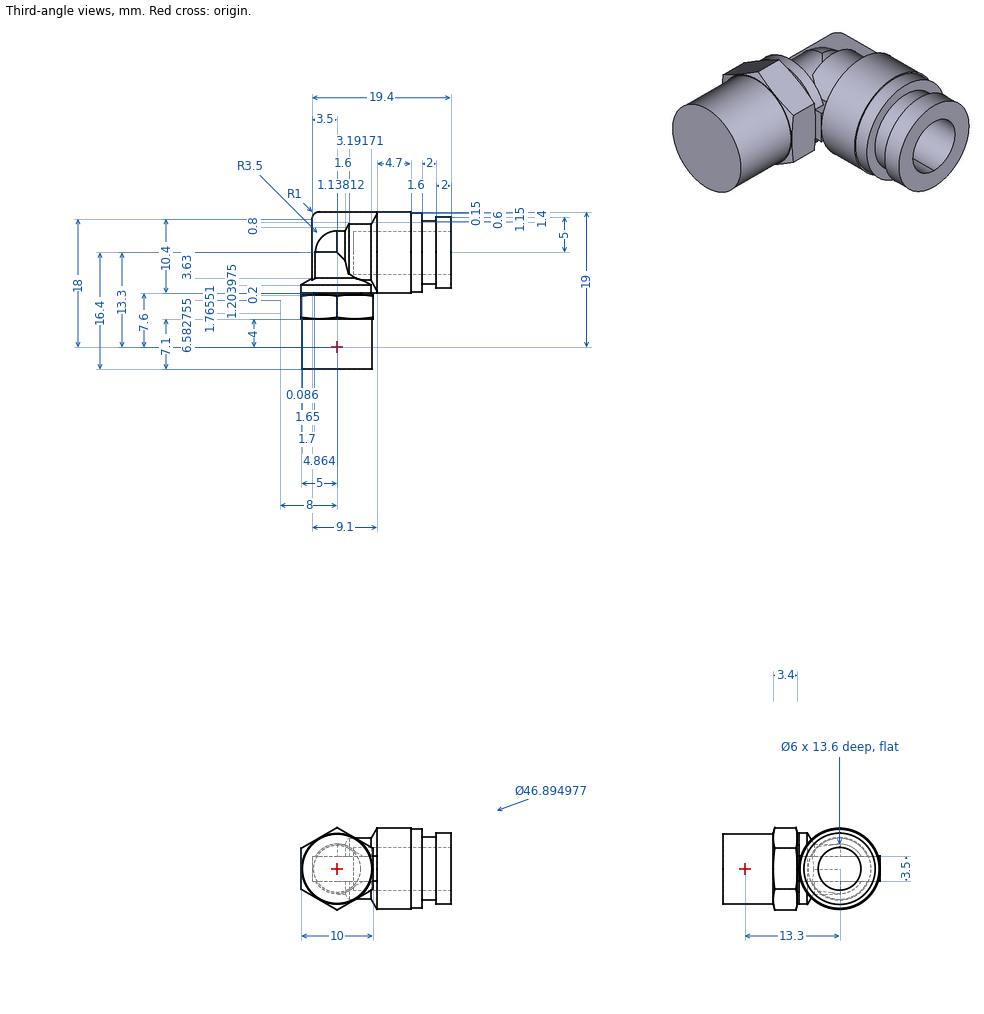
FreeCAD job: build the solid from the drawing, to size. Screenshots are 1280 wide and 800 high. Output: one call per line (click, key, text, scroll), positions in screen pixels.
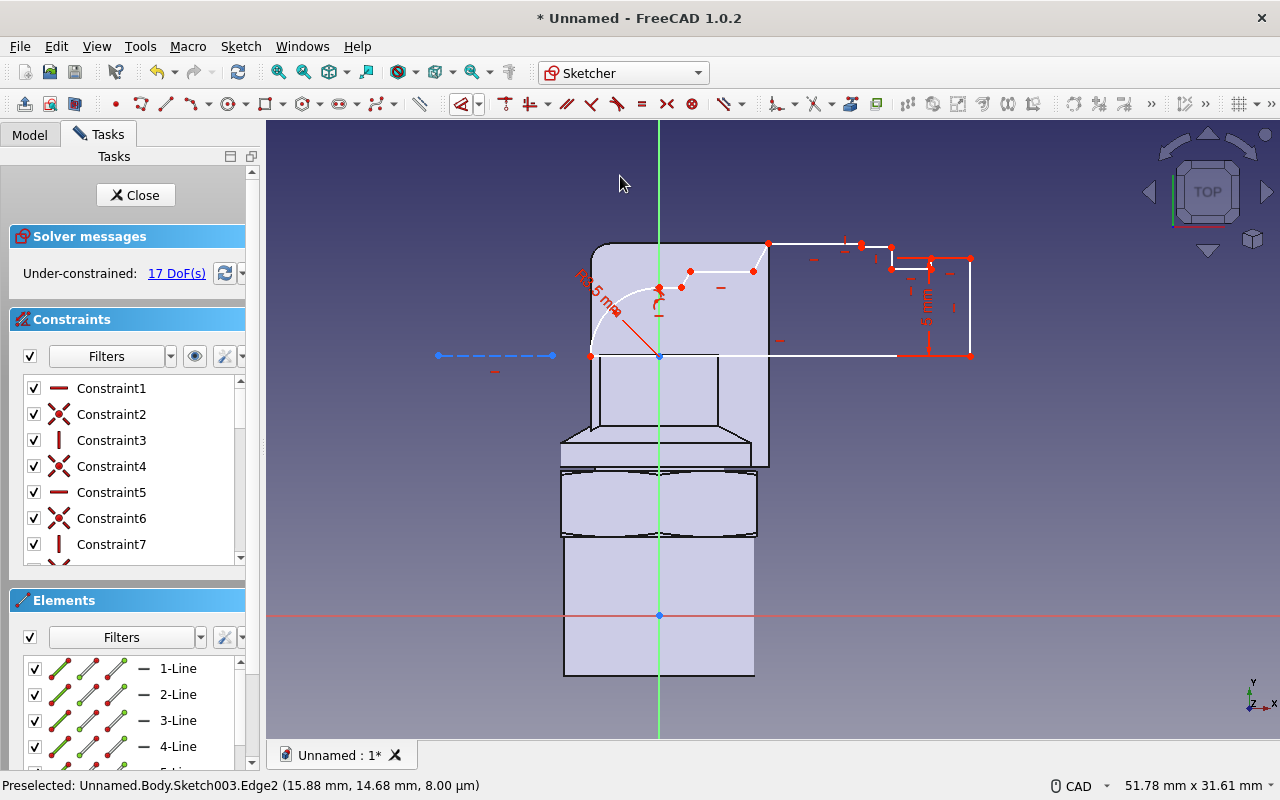
click(958, 258)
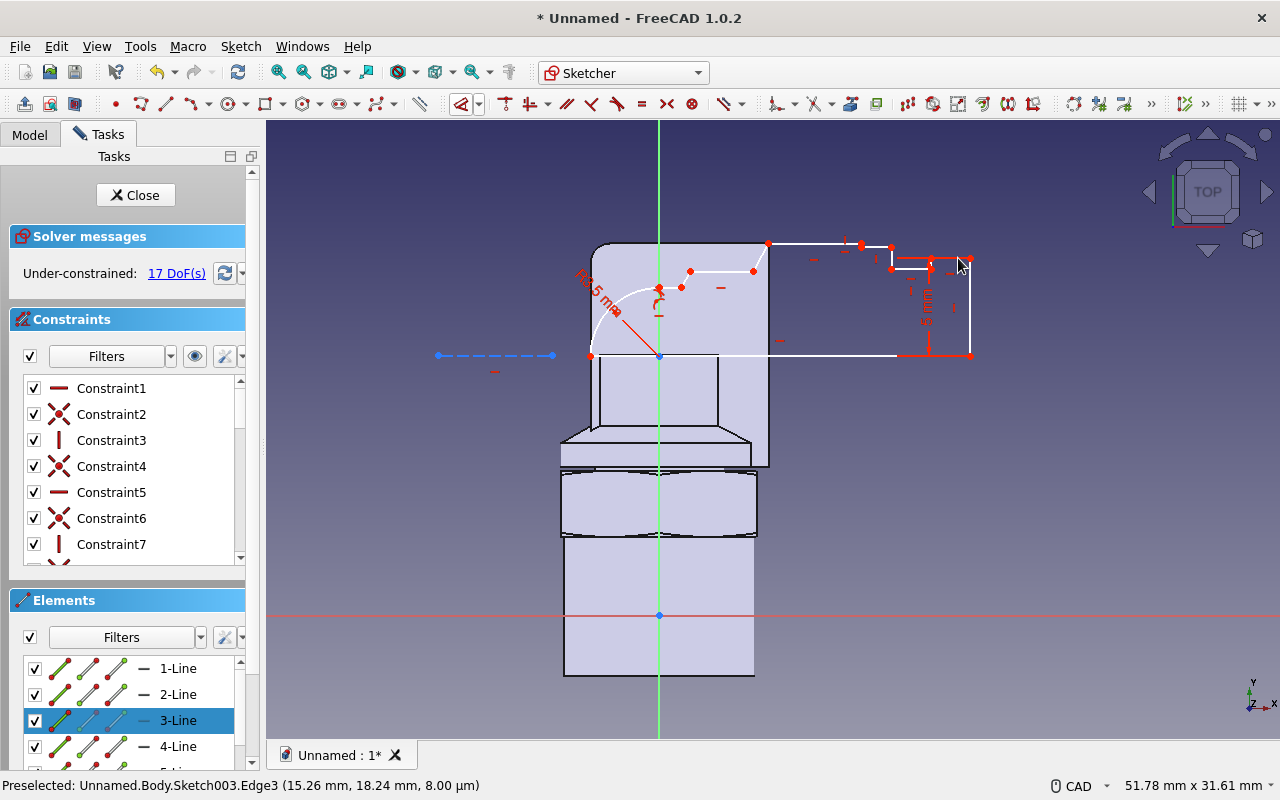
key(l)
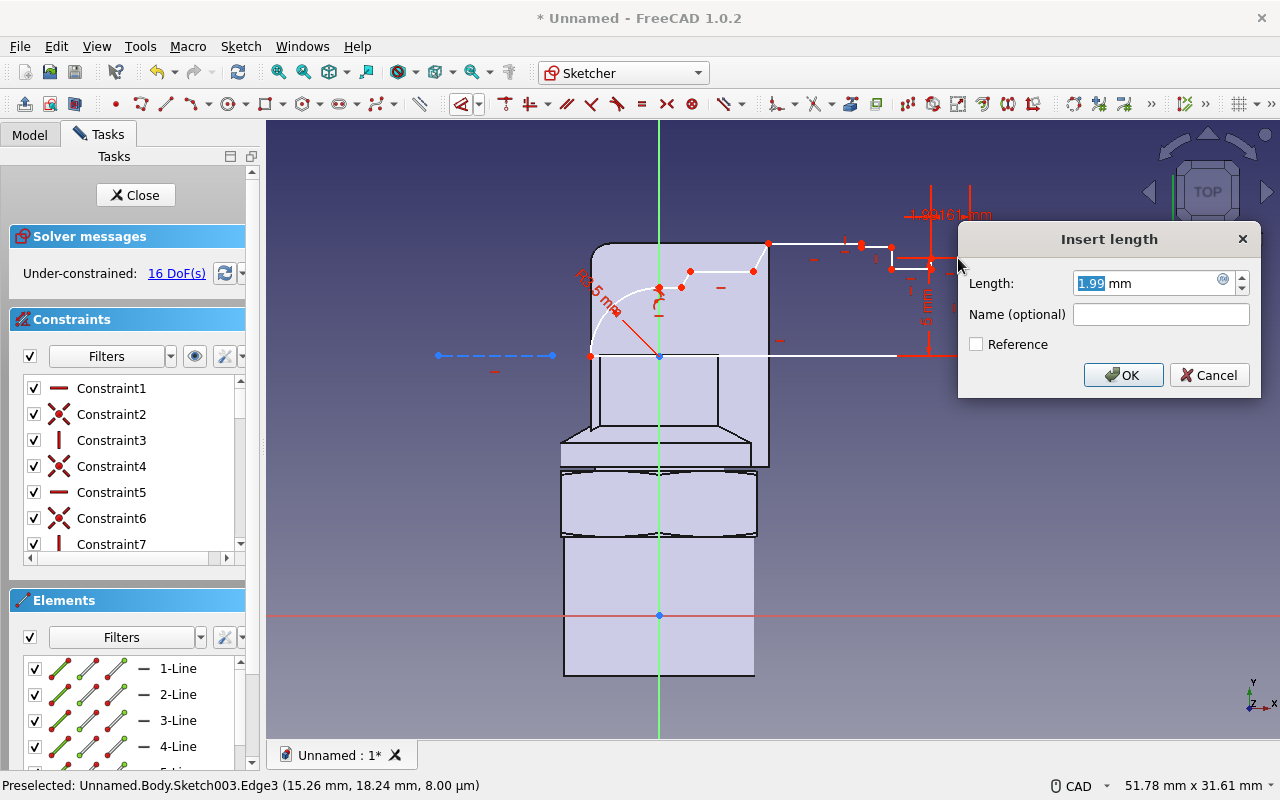
text(2)
key(Return)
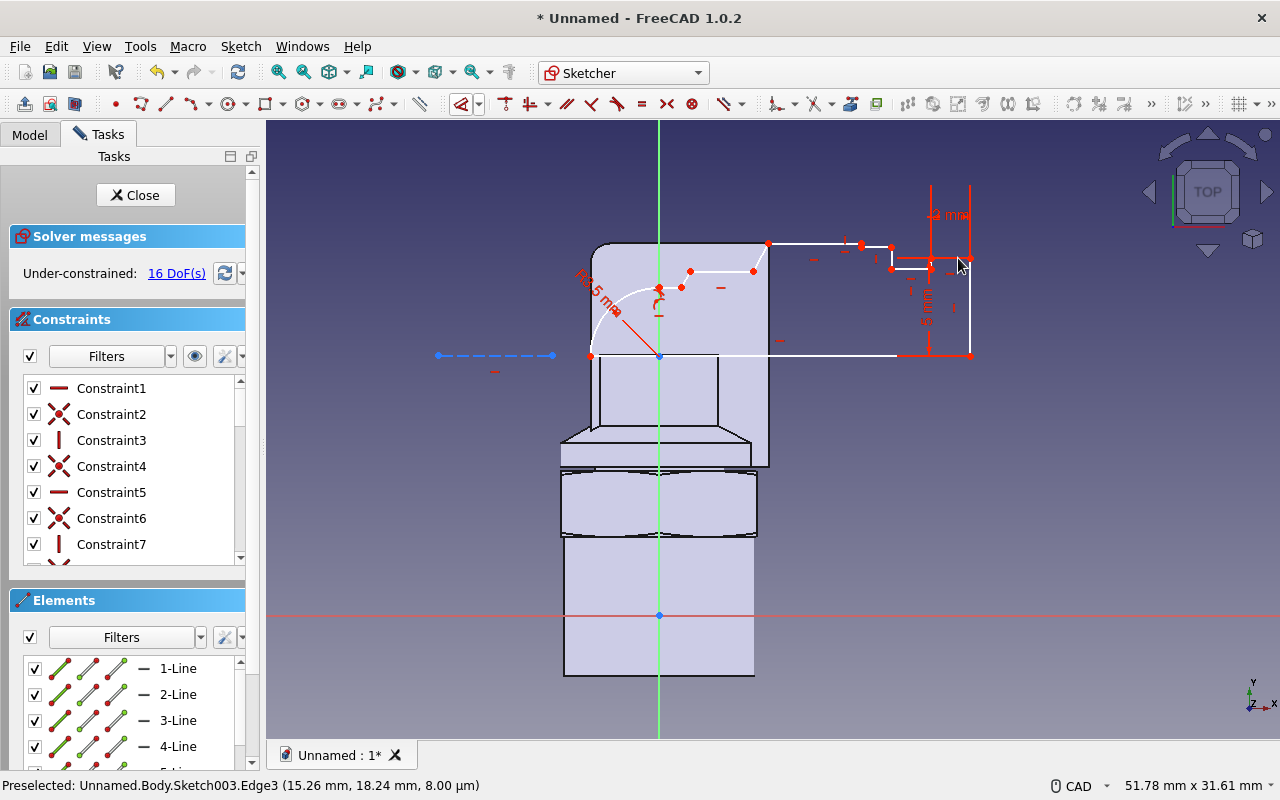
click(919, 269)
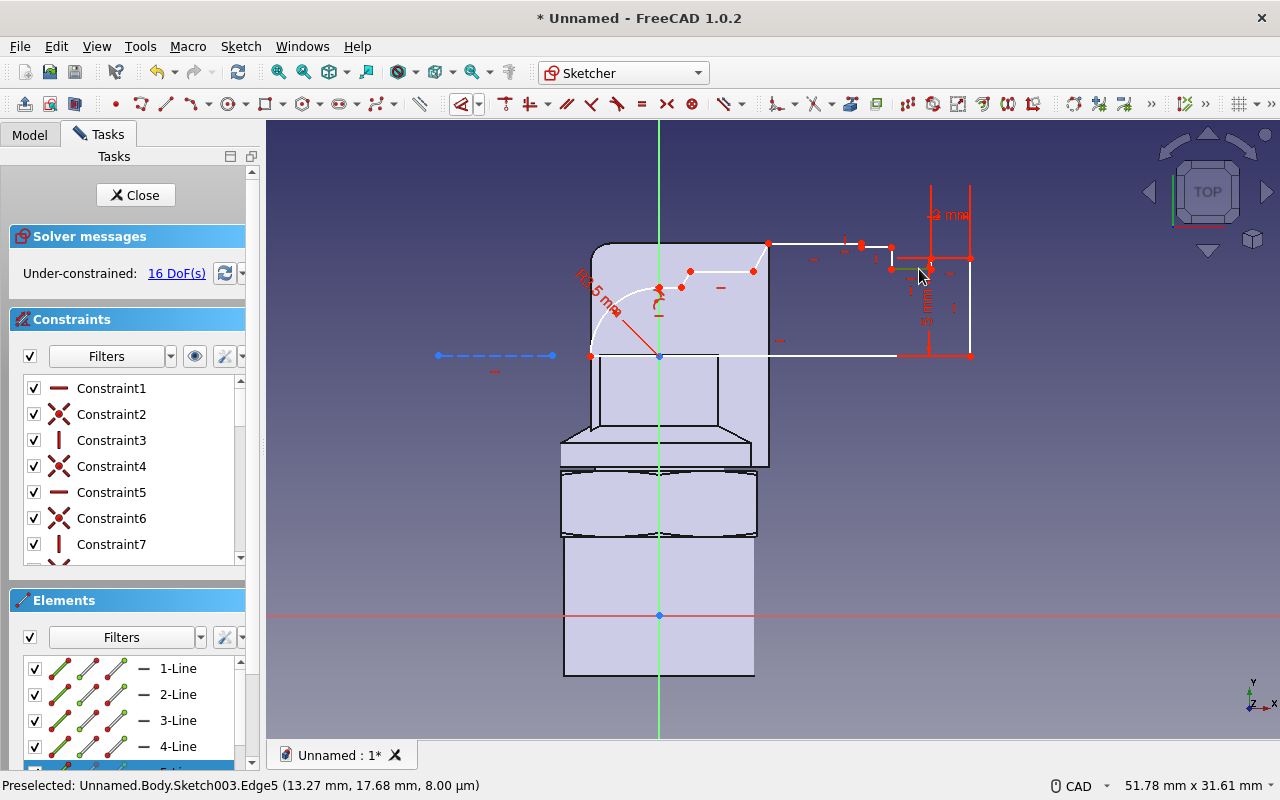
key(l)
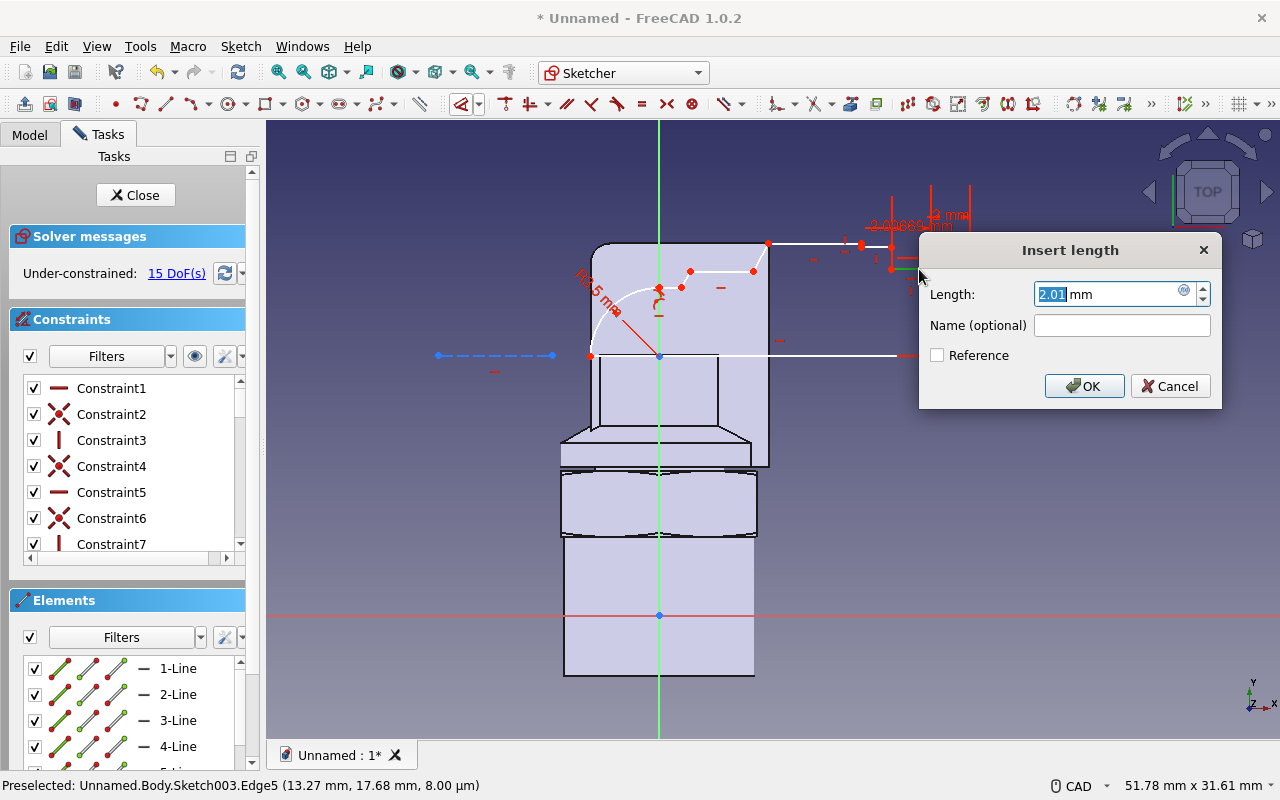
text(2)
key(Return)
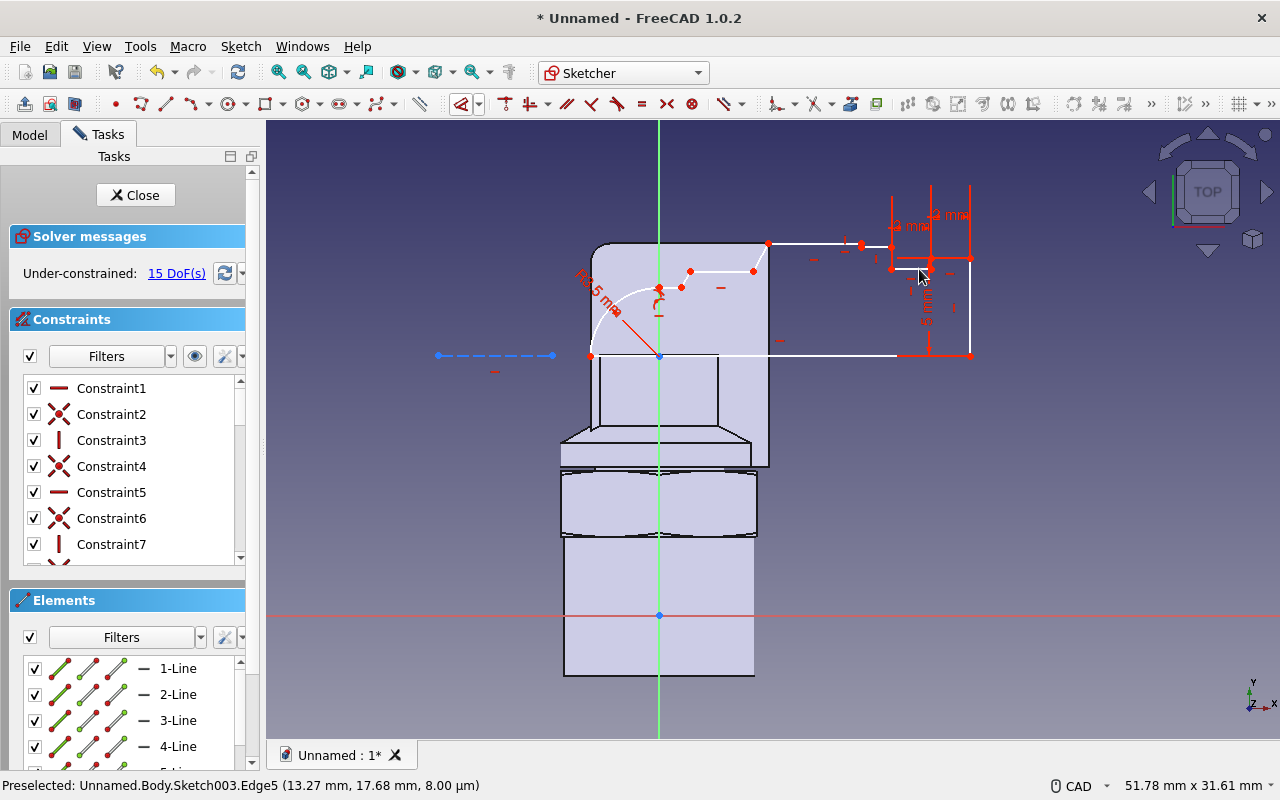
scroll(931, 264, up, 7)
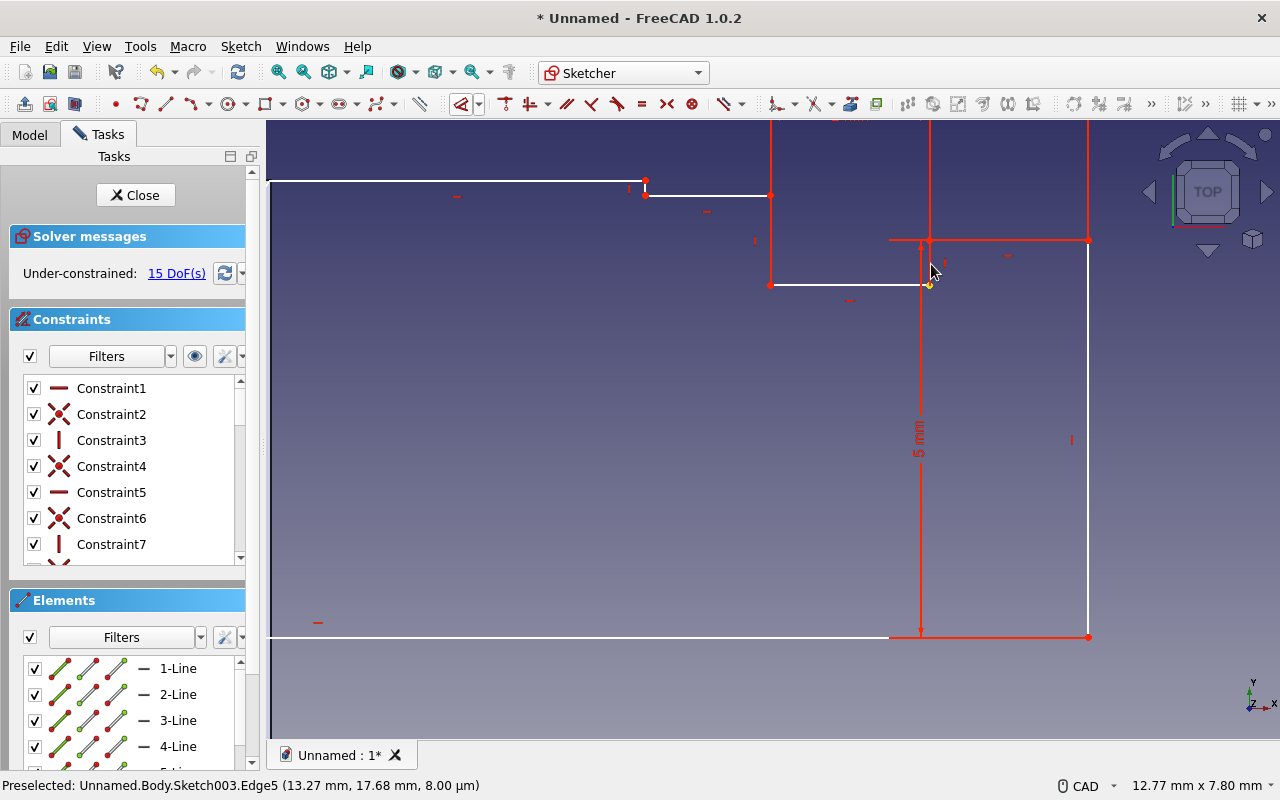
click(930, 263)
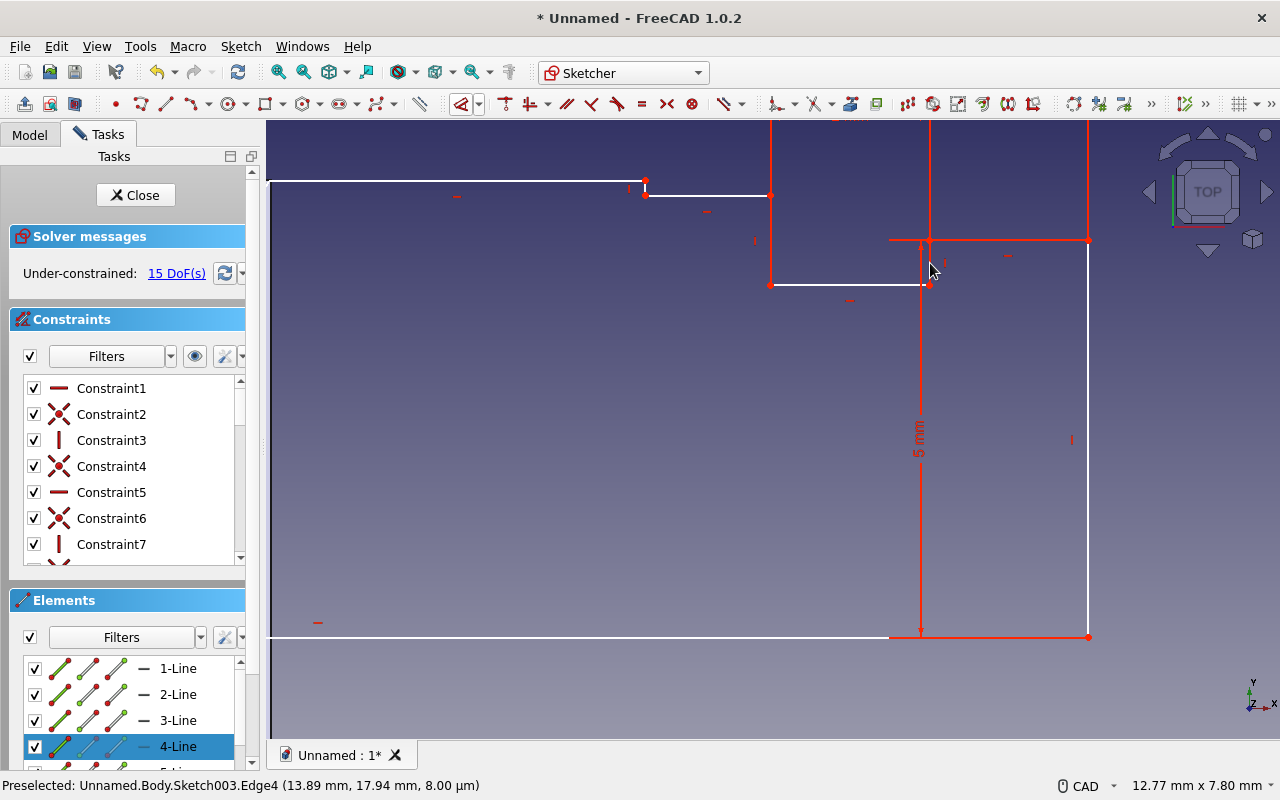
key(i)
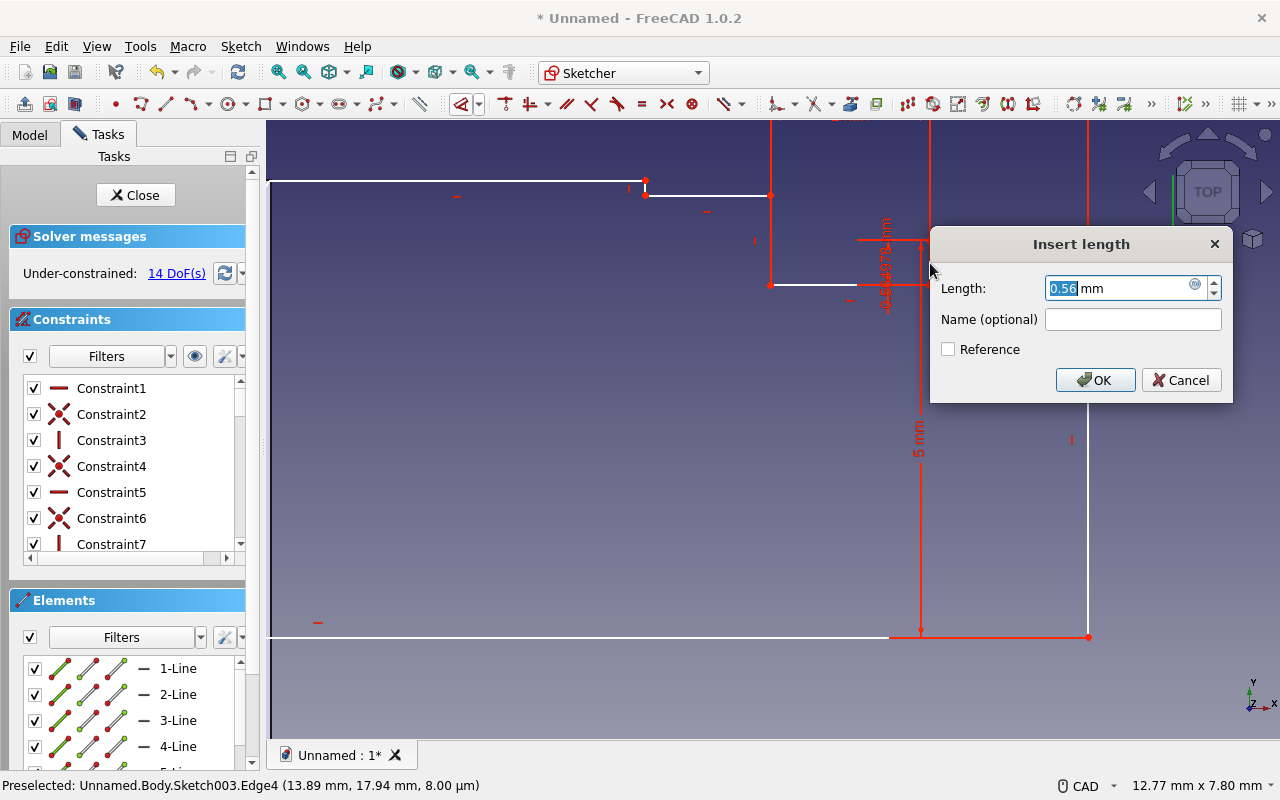
text(0.6)
key(Return)